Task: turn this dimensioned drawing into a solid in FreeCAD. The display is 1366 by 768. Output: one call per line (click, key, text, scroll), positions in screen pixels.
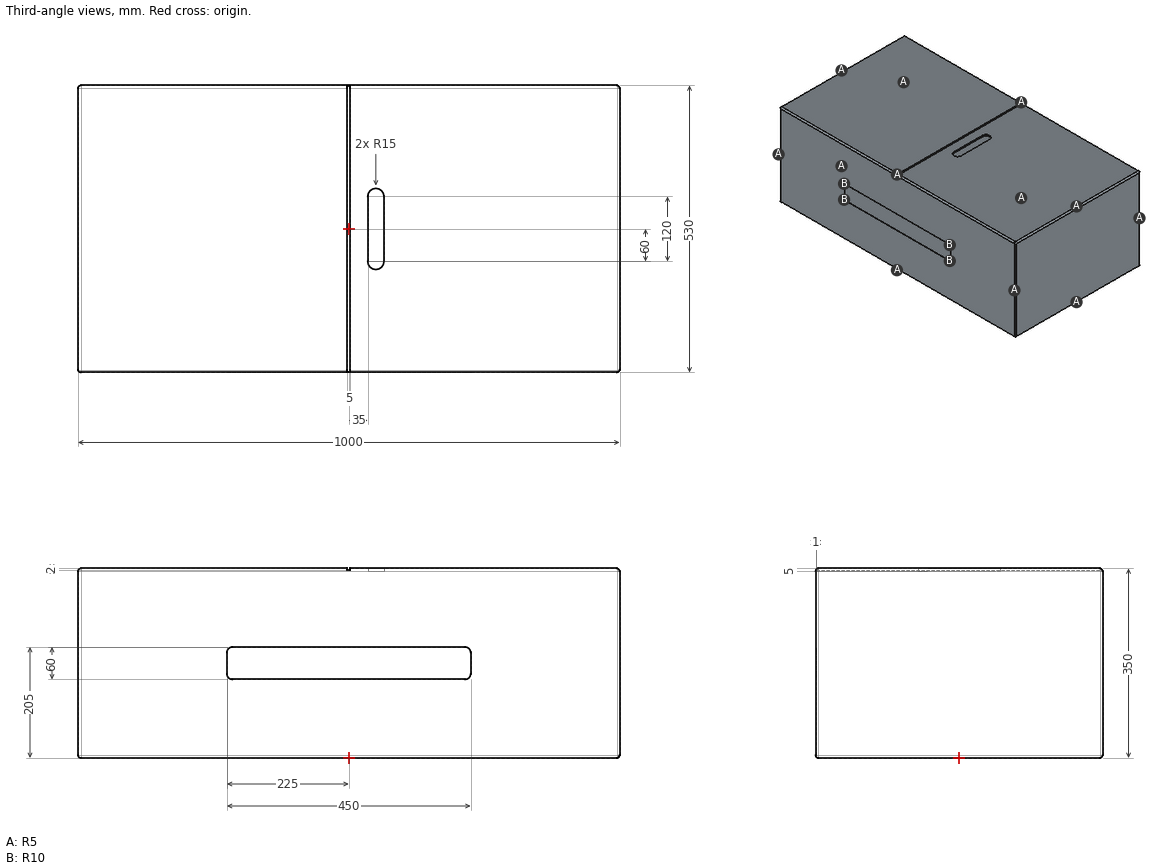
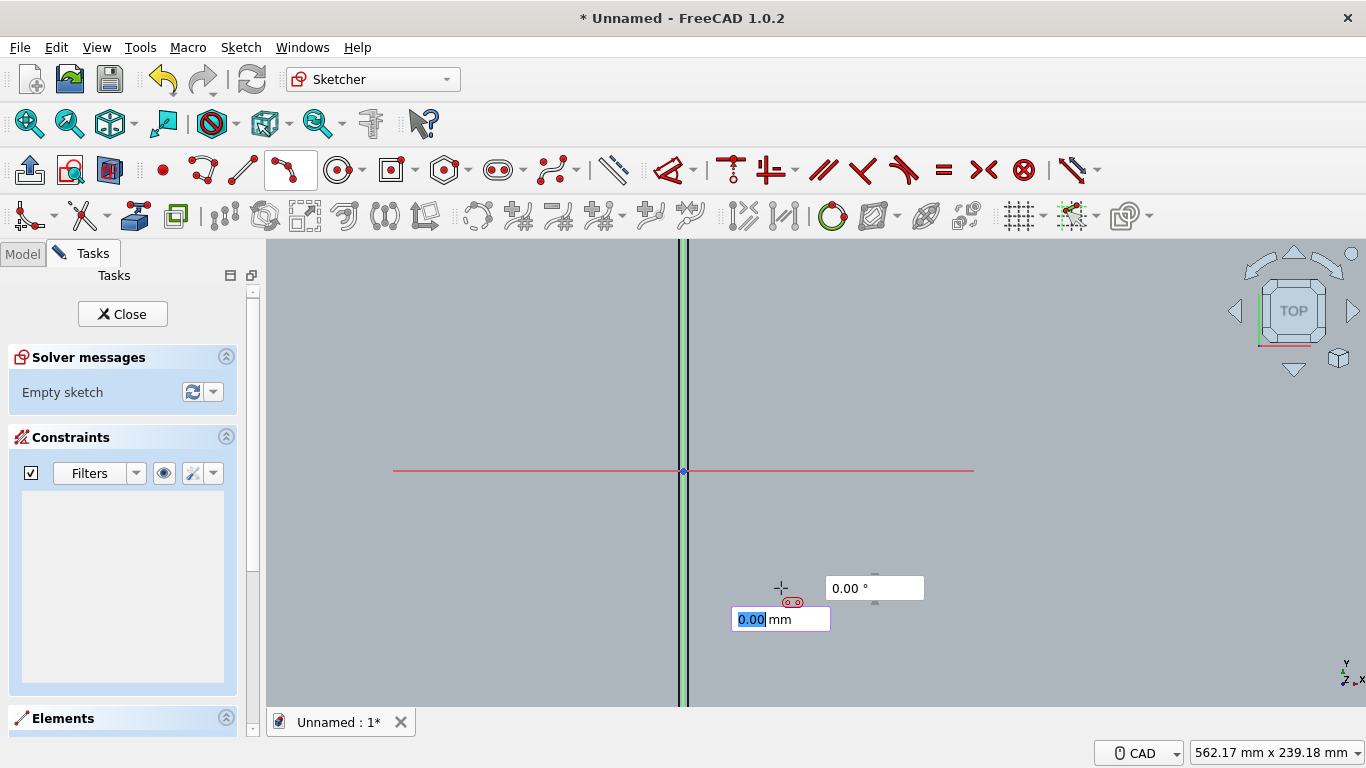
click(781, 354)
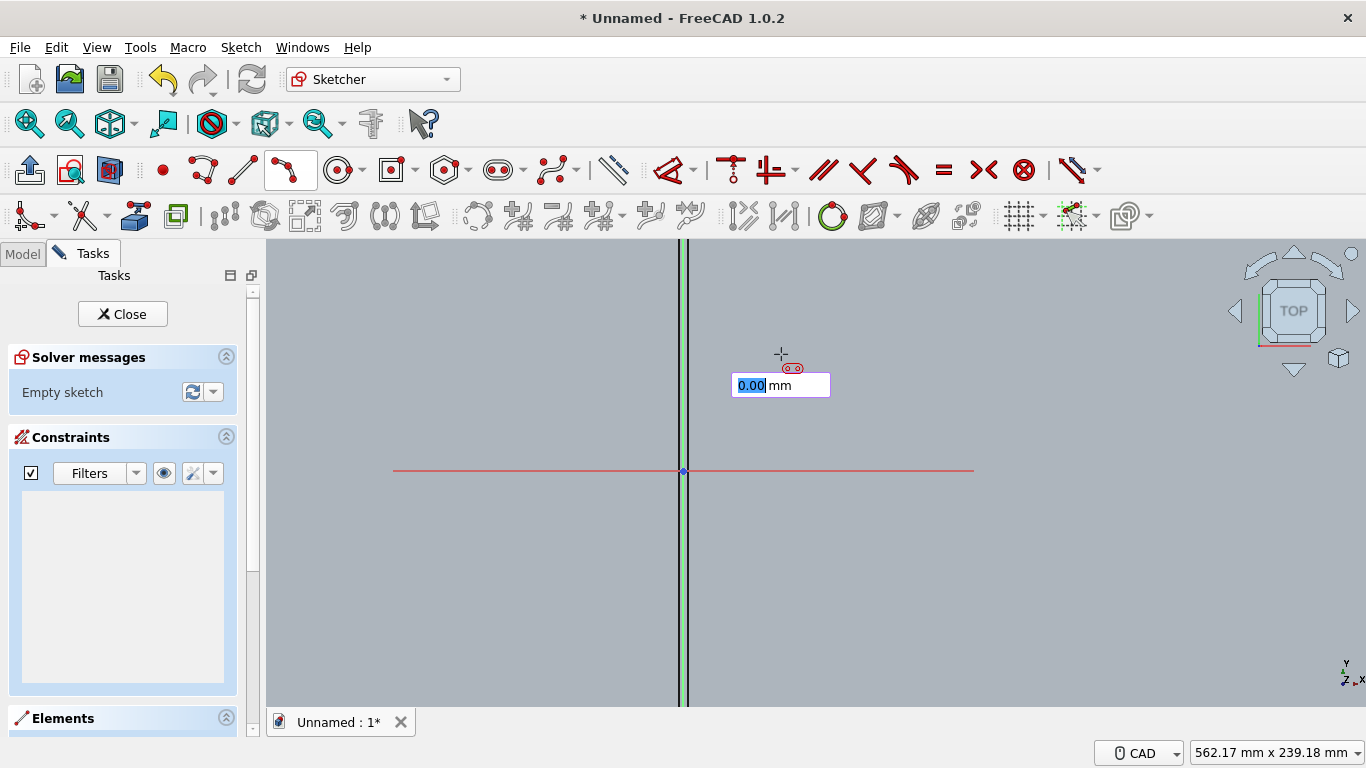
click(811, 506)
key(Escape)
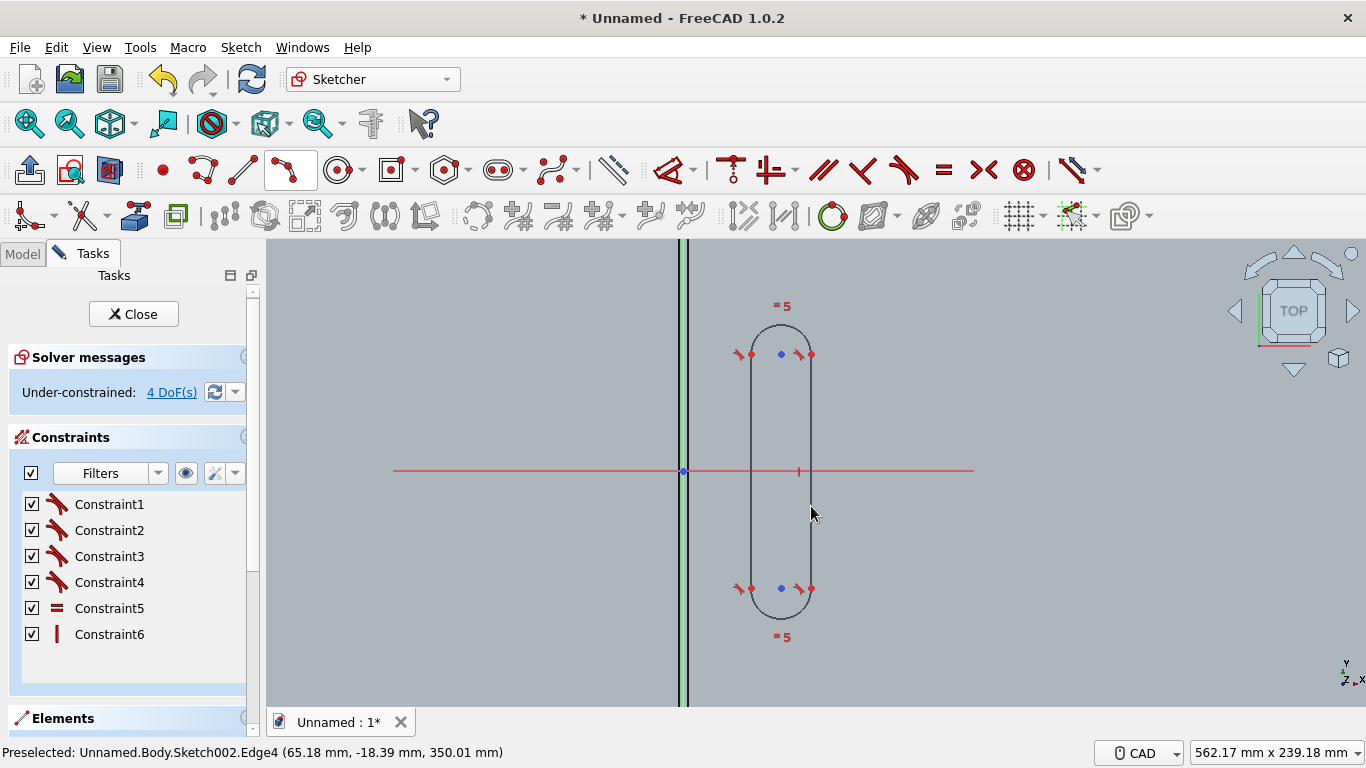
click(668, 170)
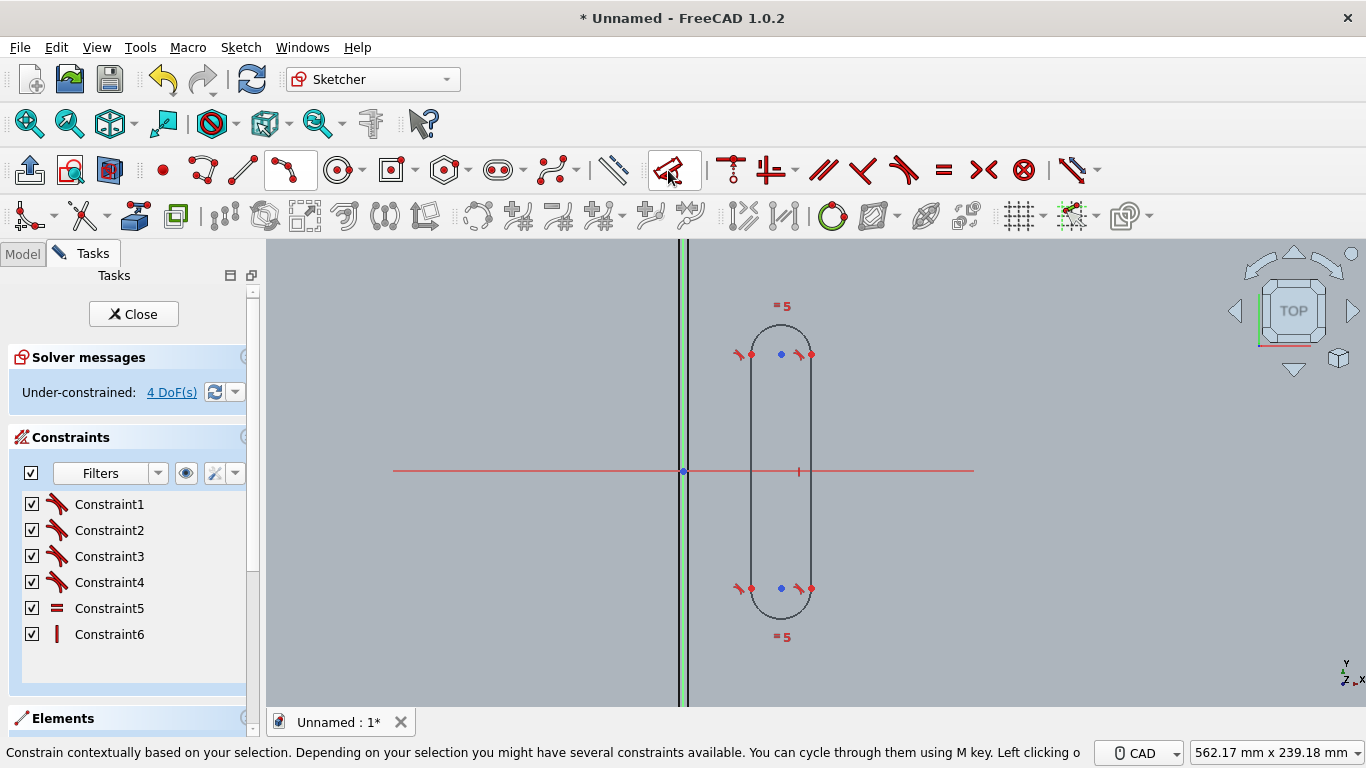
scroll(763, 613, up, 2)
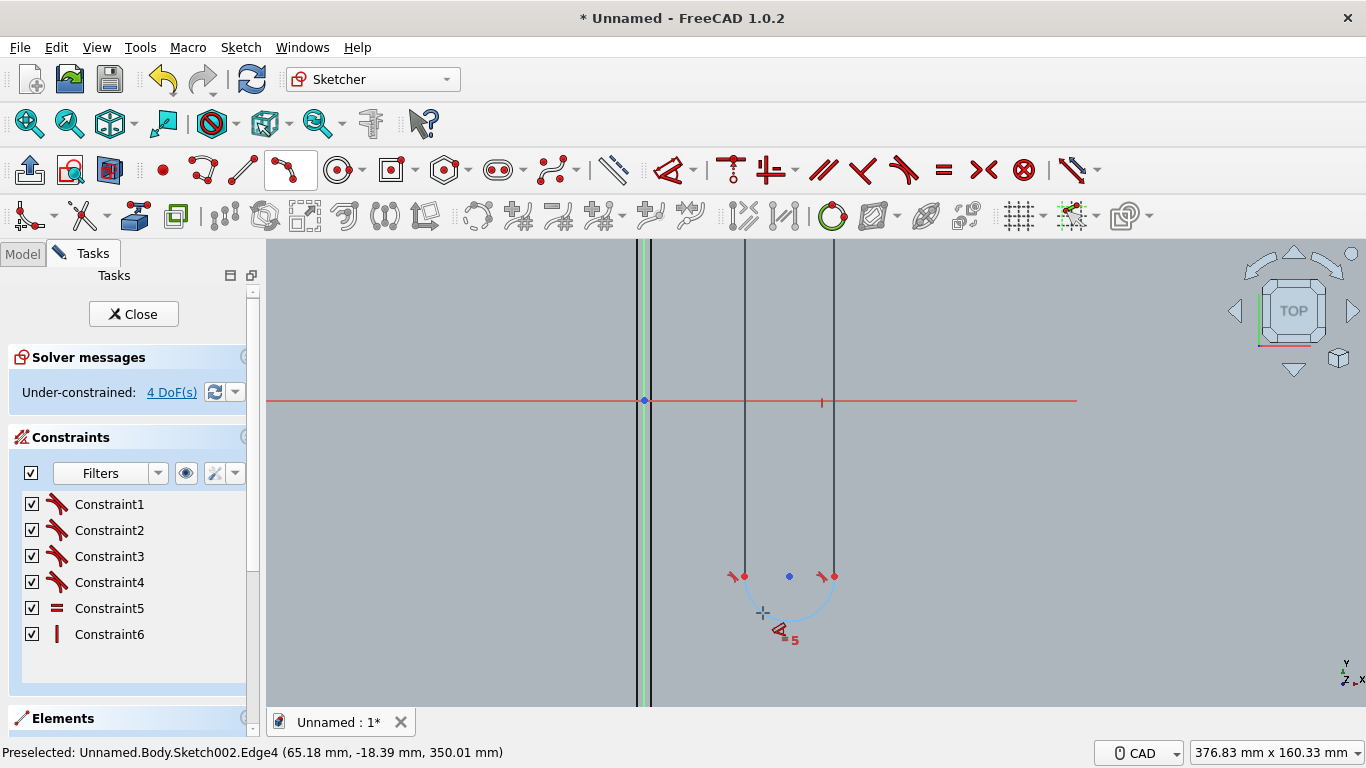
click(763, 613)
click(744, 639)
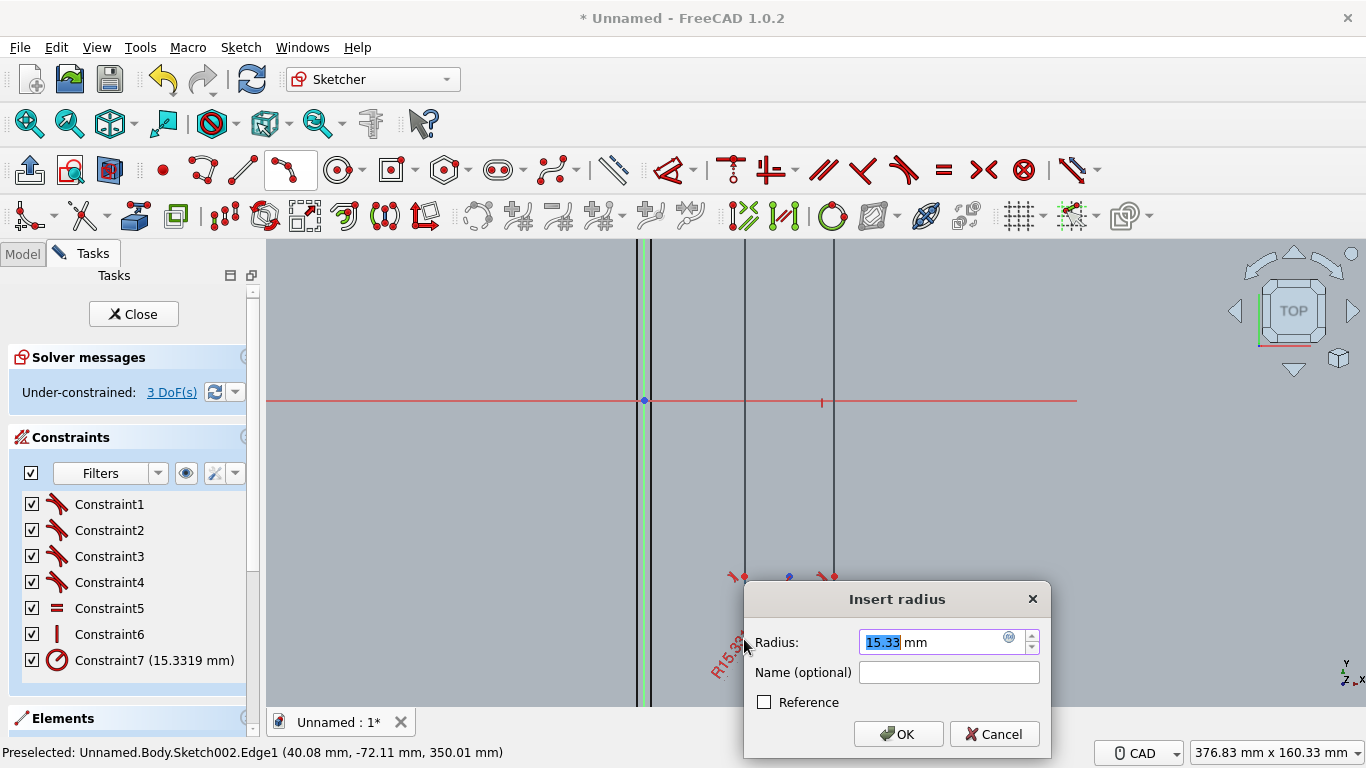
text(15)
key(Return)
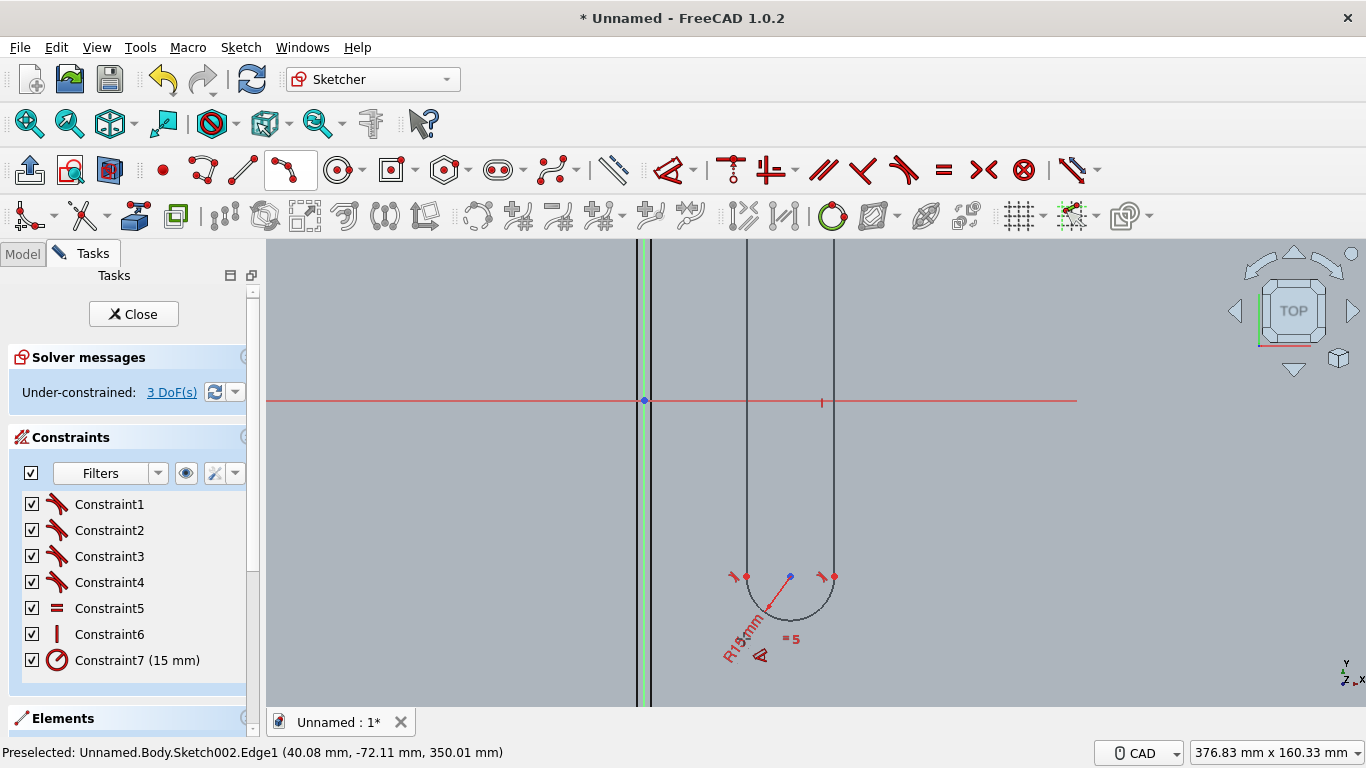
click(747, 472)
click(781, 422)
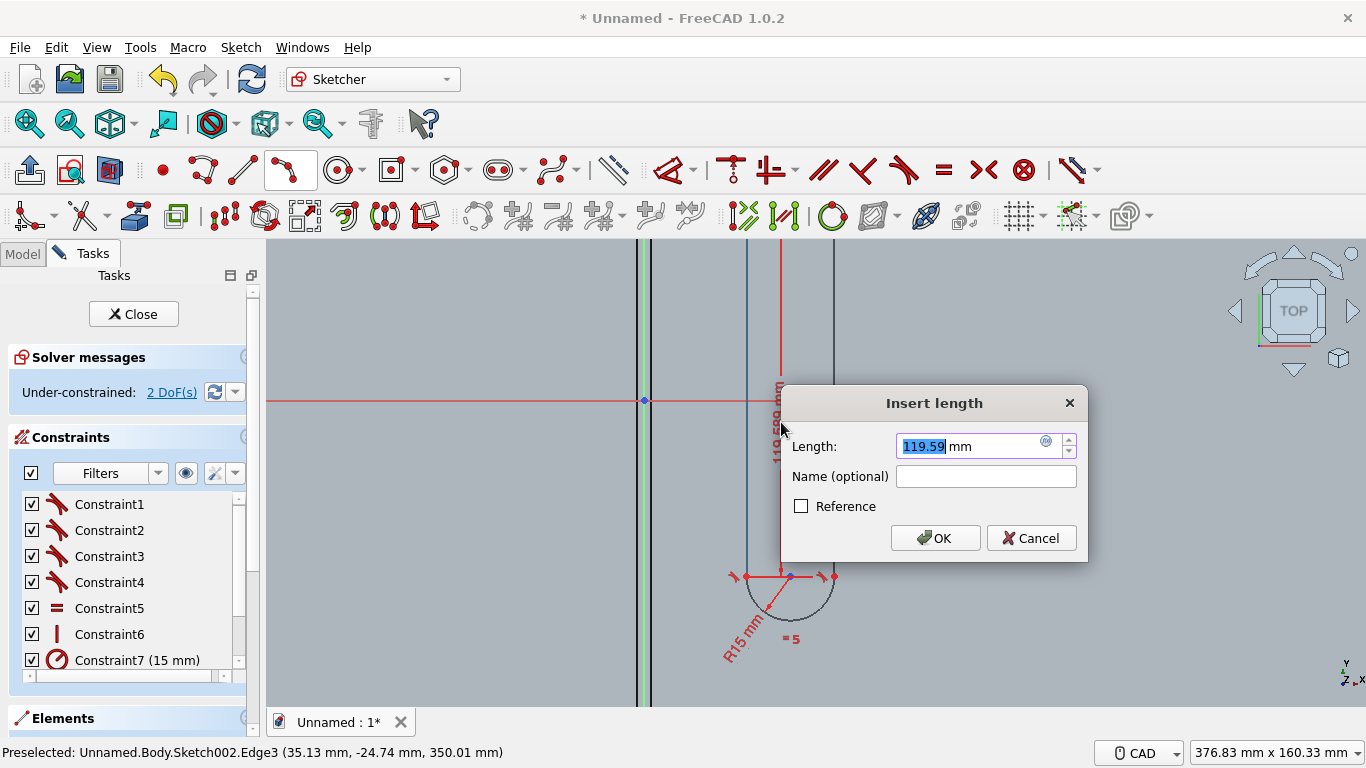
text(120)
key(Return)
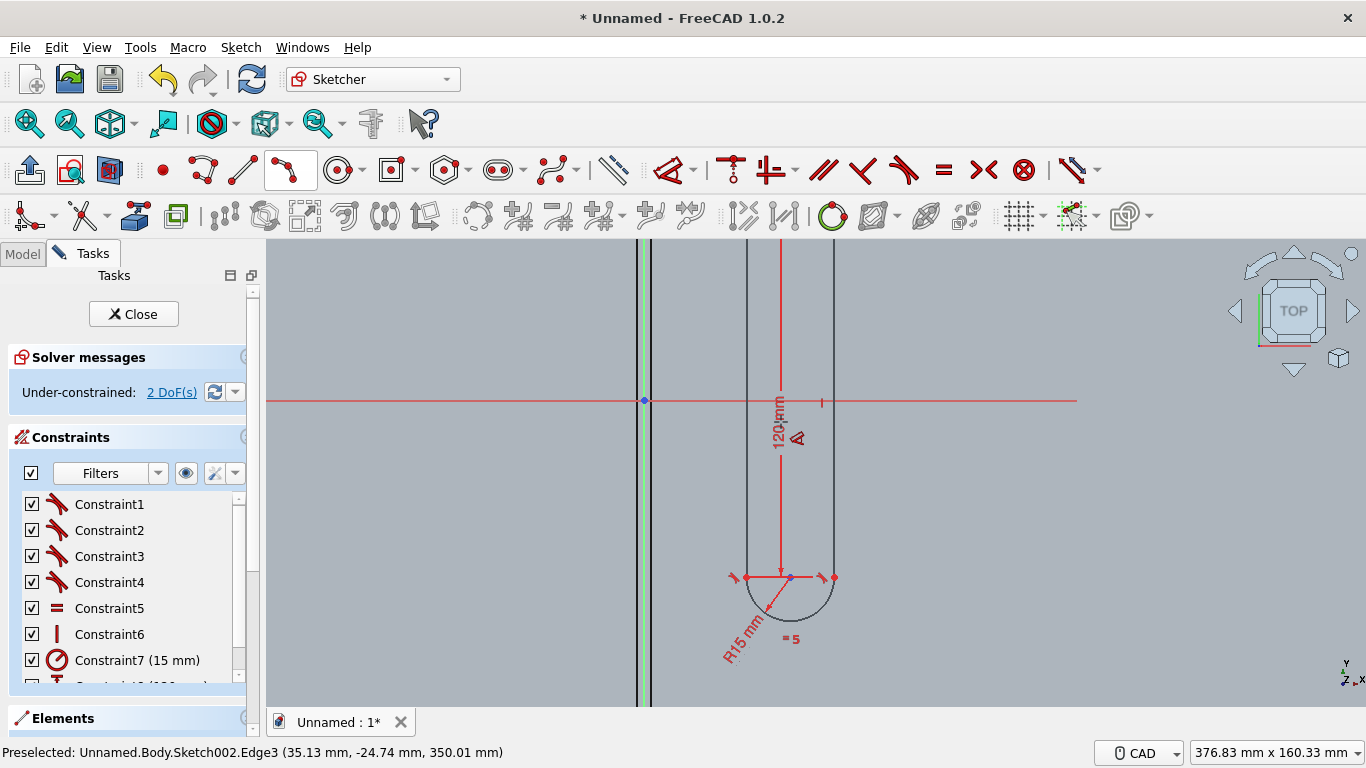
click(747, 577)
click(695, 611)